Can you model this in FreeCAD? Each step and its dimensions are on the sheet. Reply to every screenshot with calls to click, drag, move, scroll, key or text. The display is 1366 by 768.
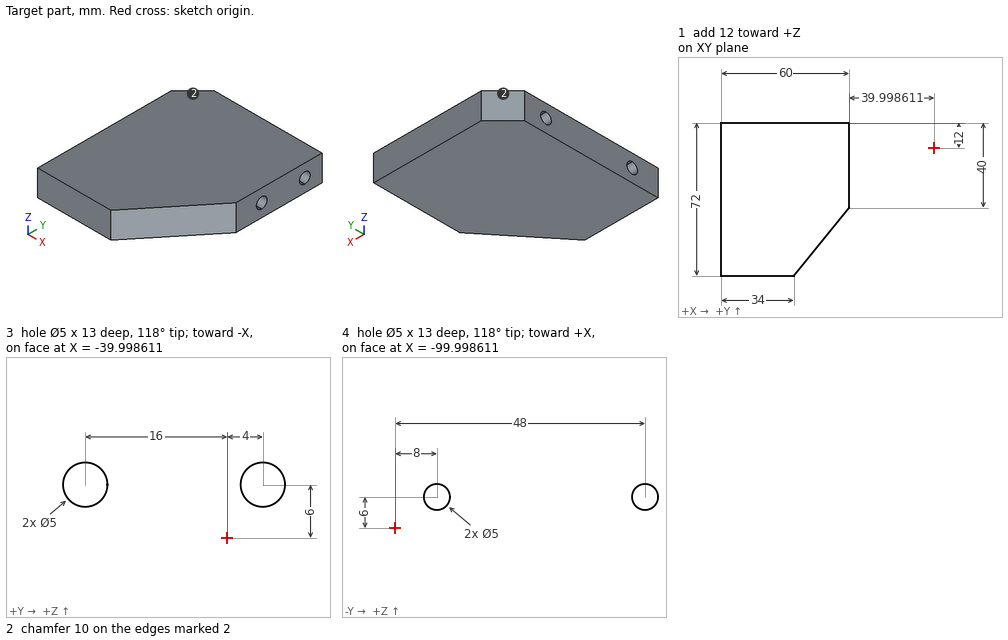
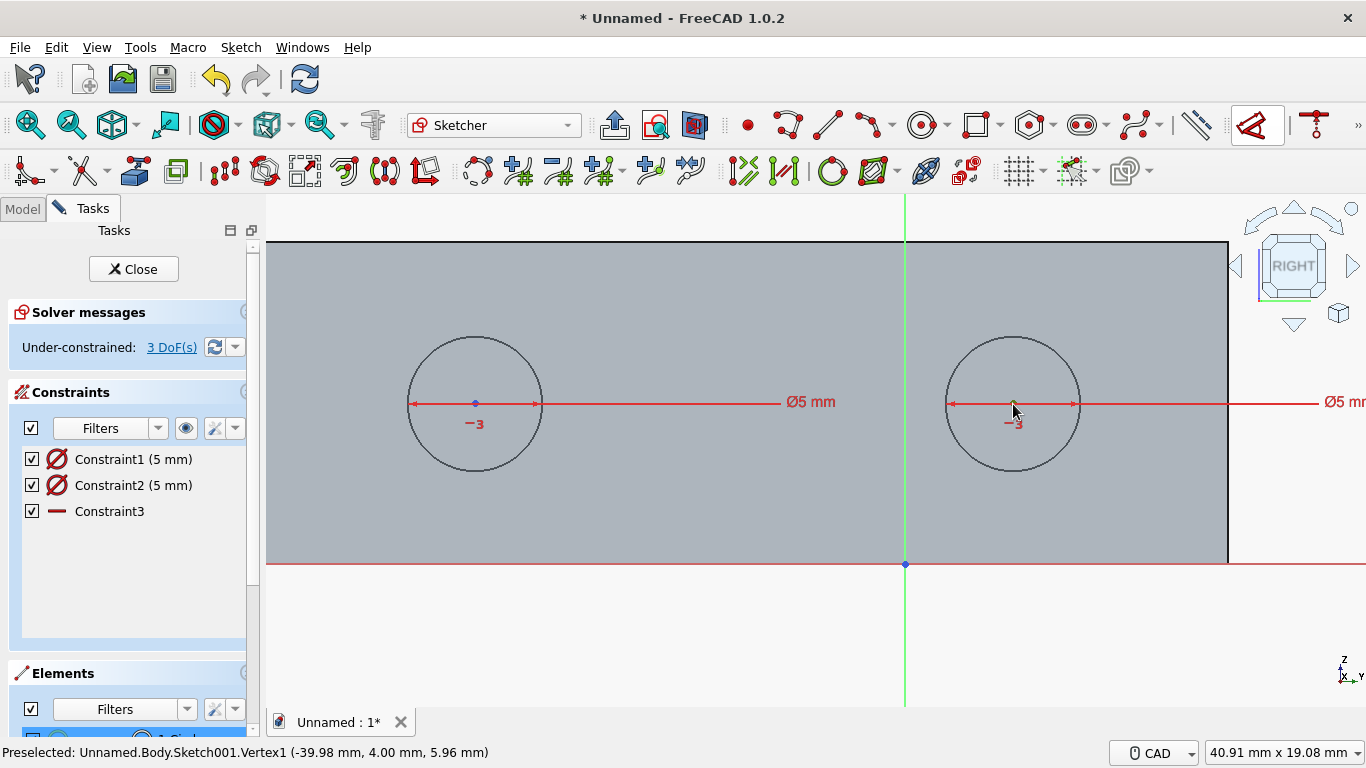
click(1278, 126)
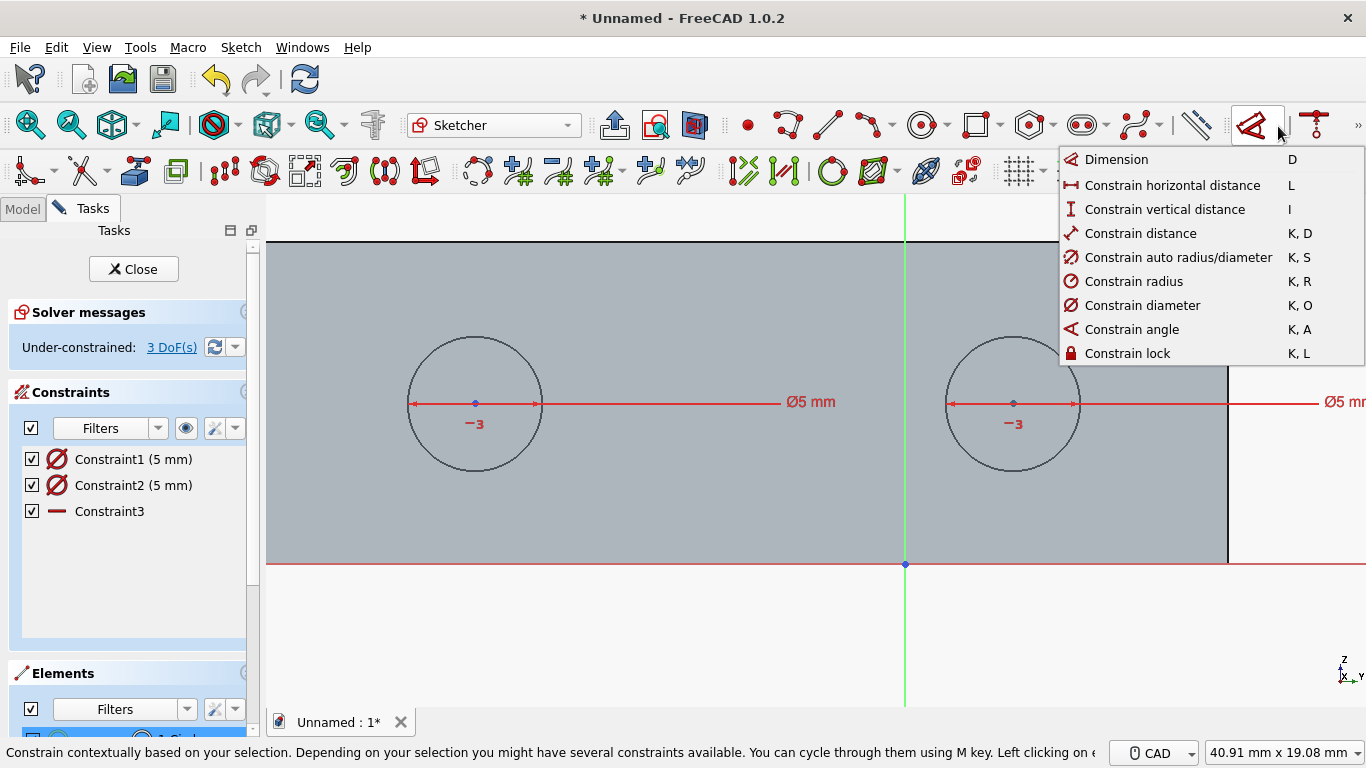
click(1212, 185)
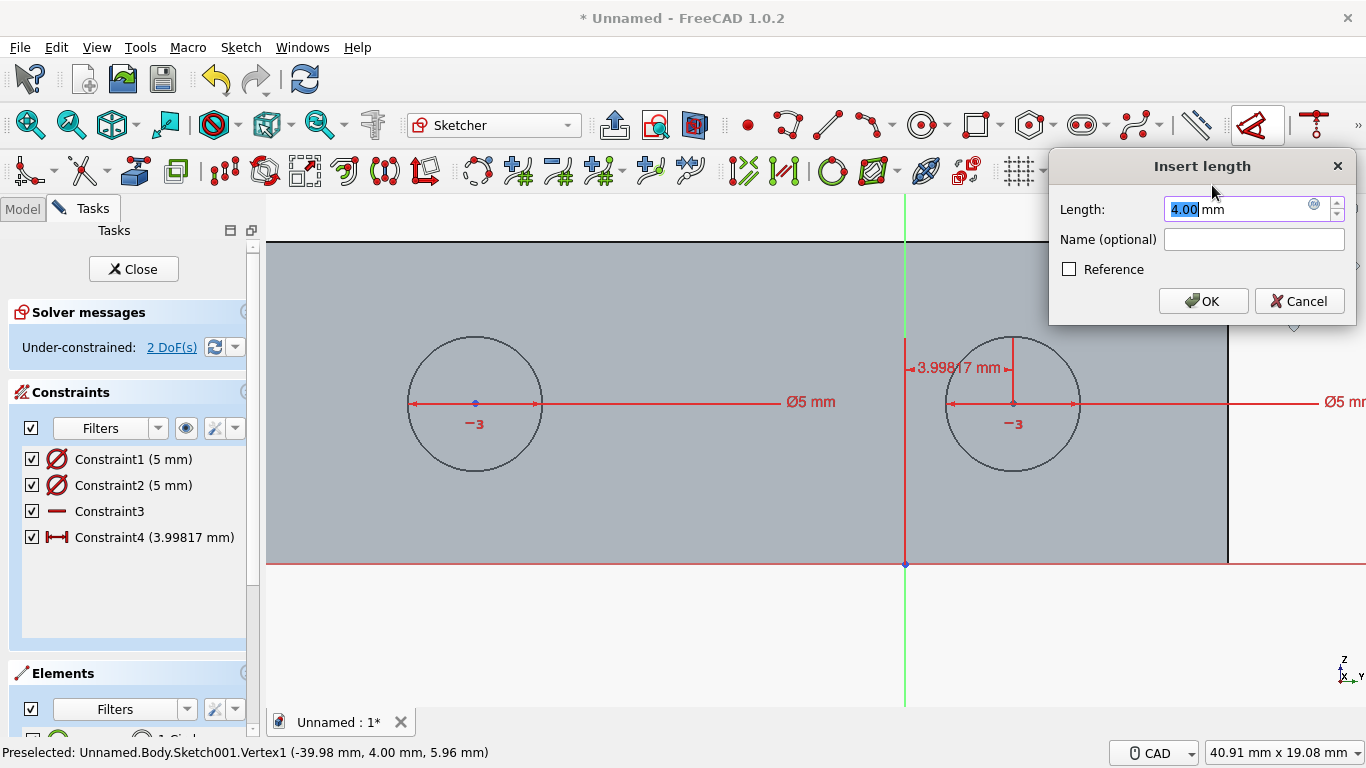
text(4)
key(Return)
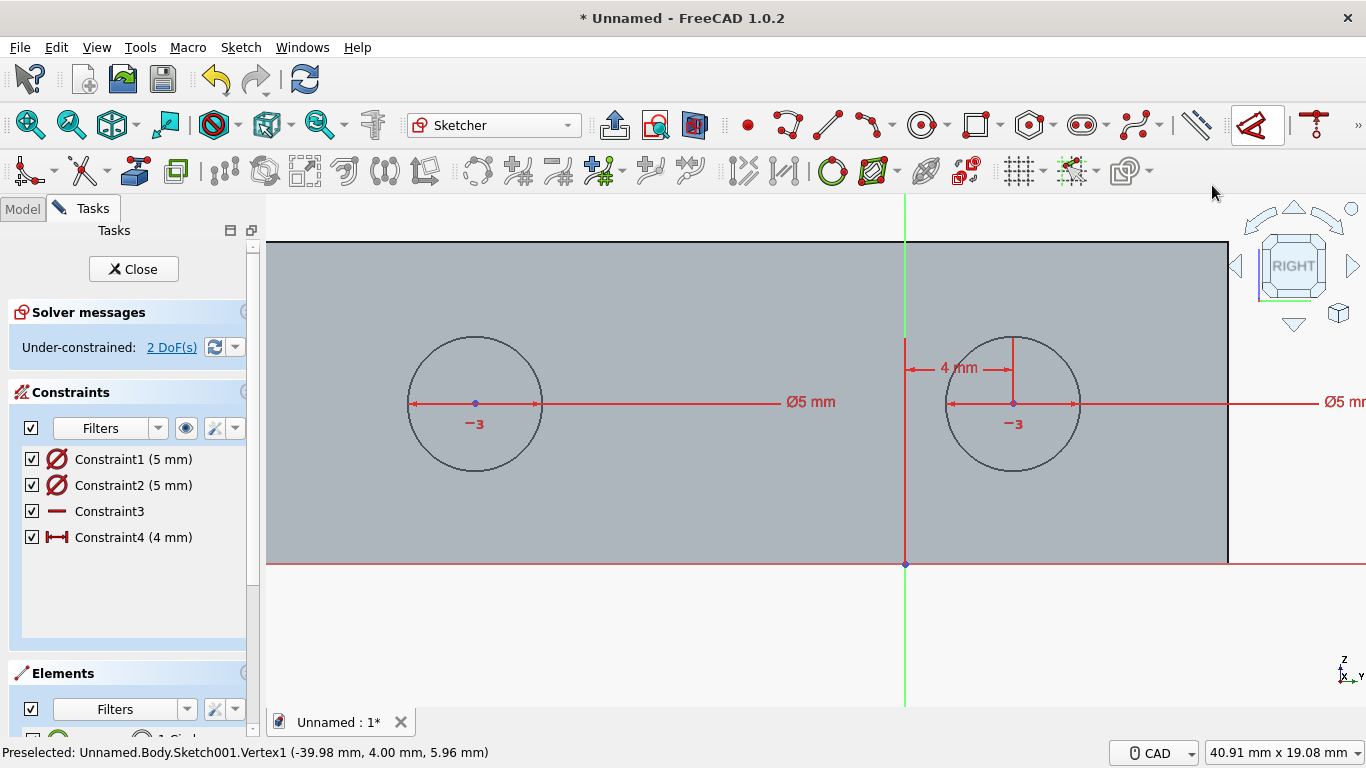
click(1013, 404)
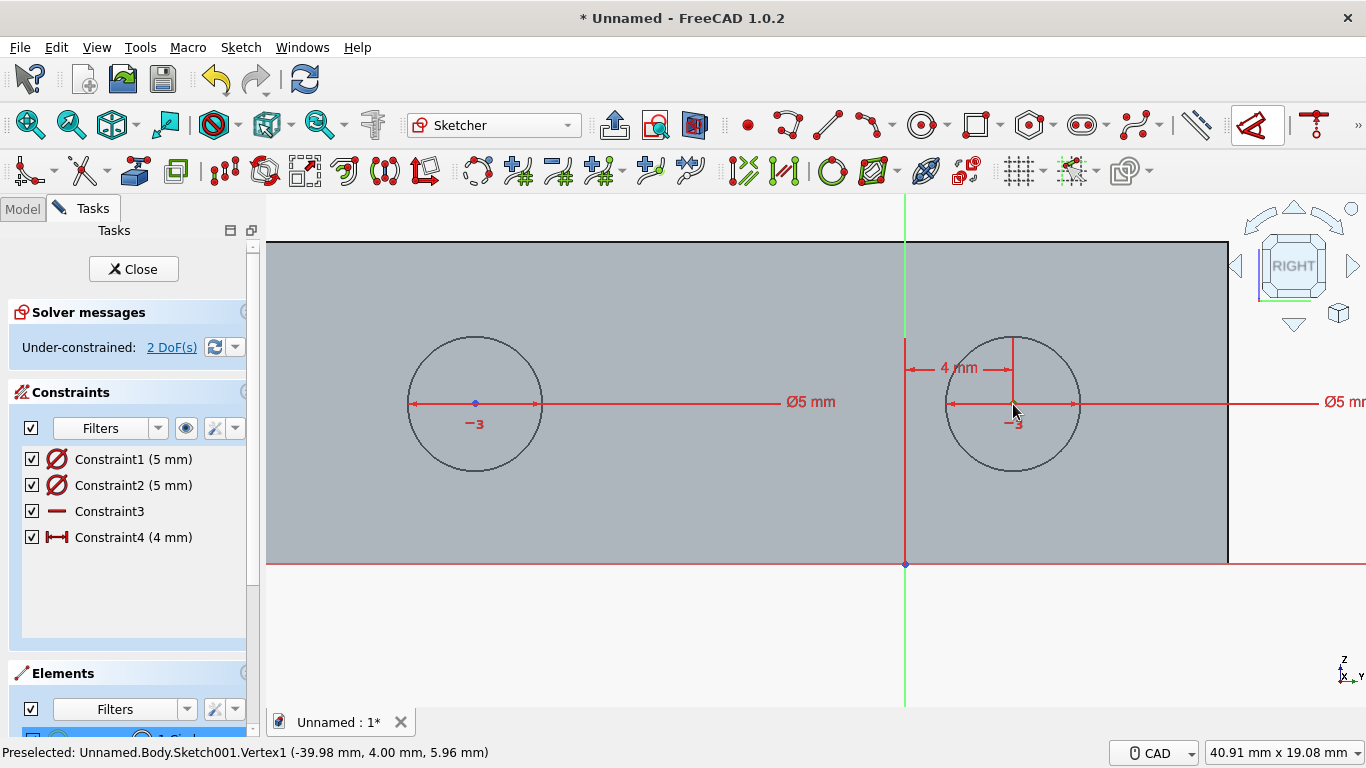
click(1278, 126)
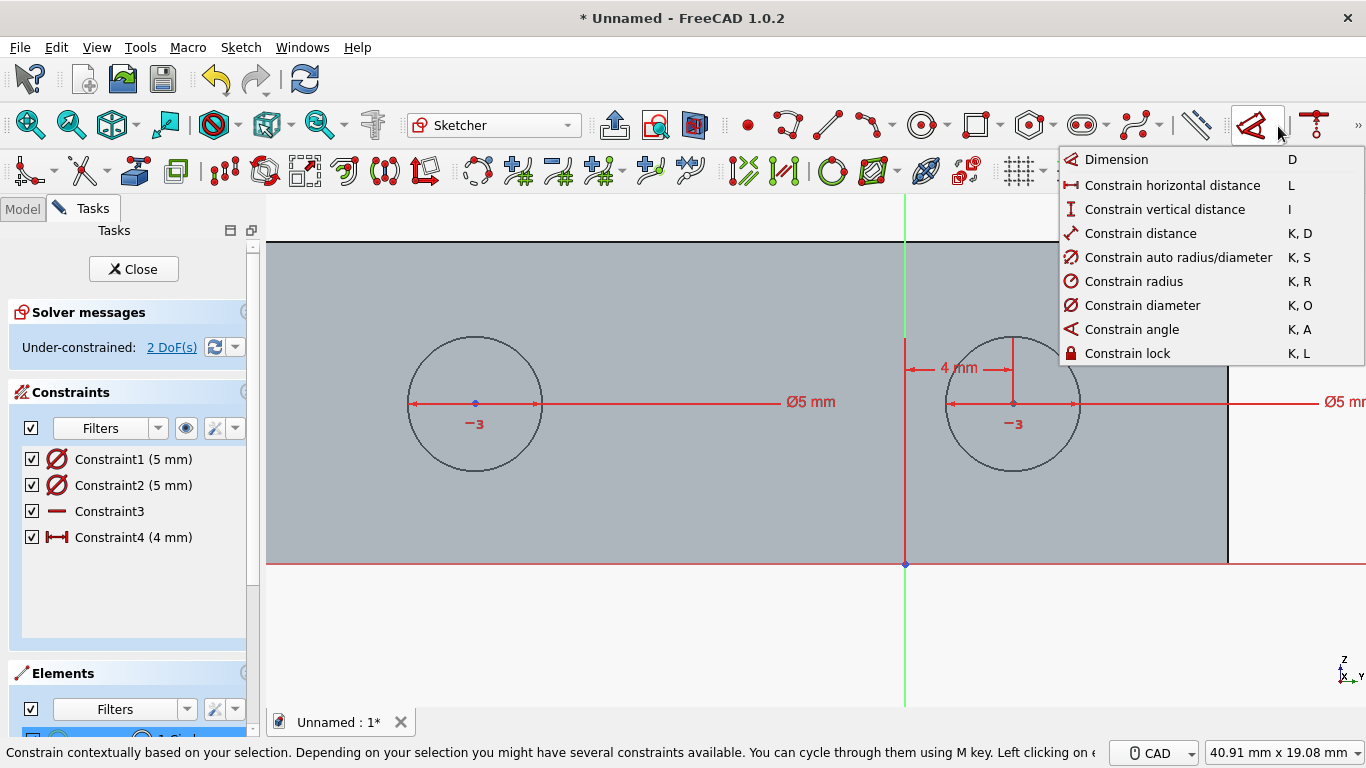
click(1212, 209)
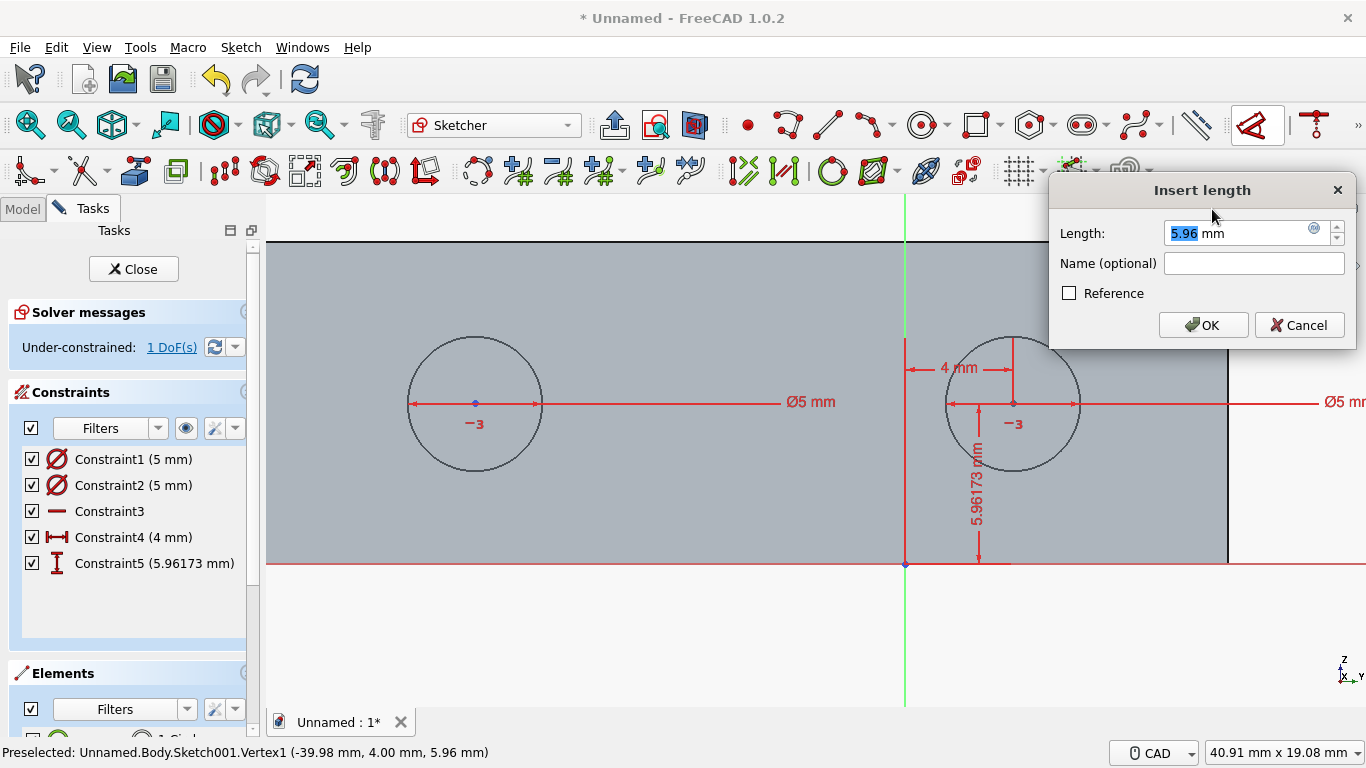
text(6)
key(Return)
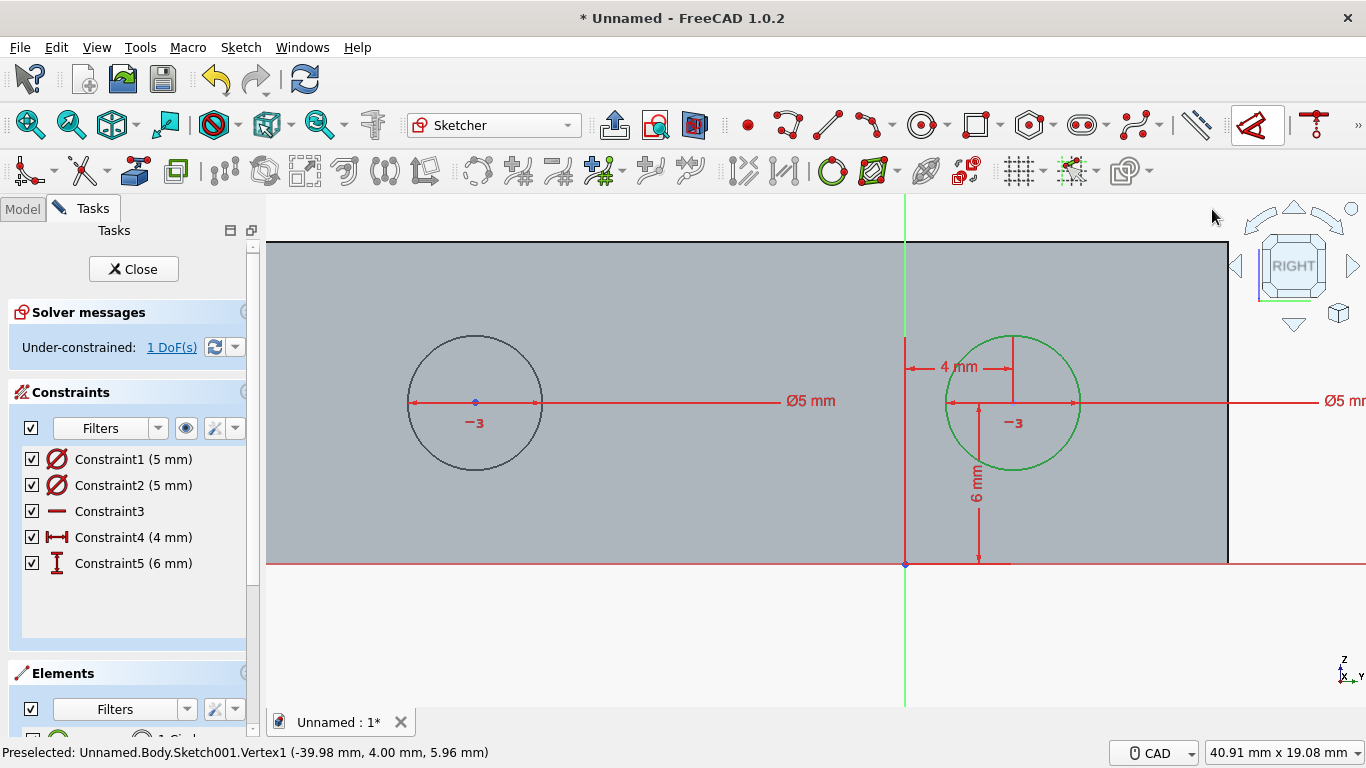
click(475, 403)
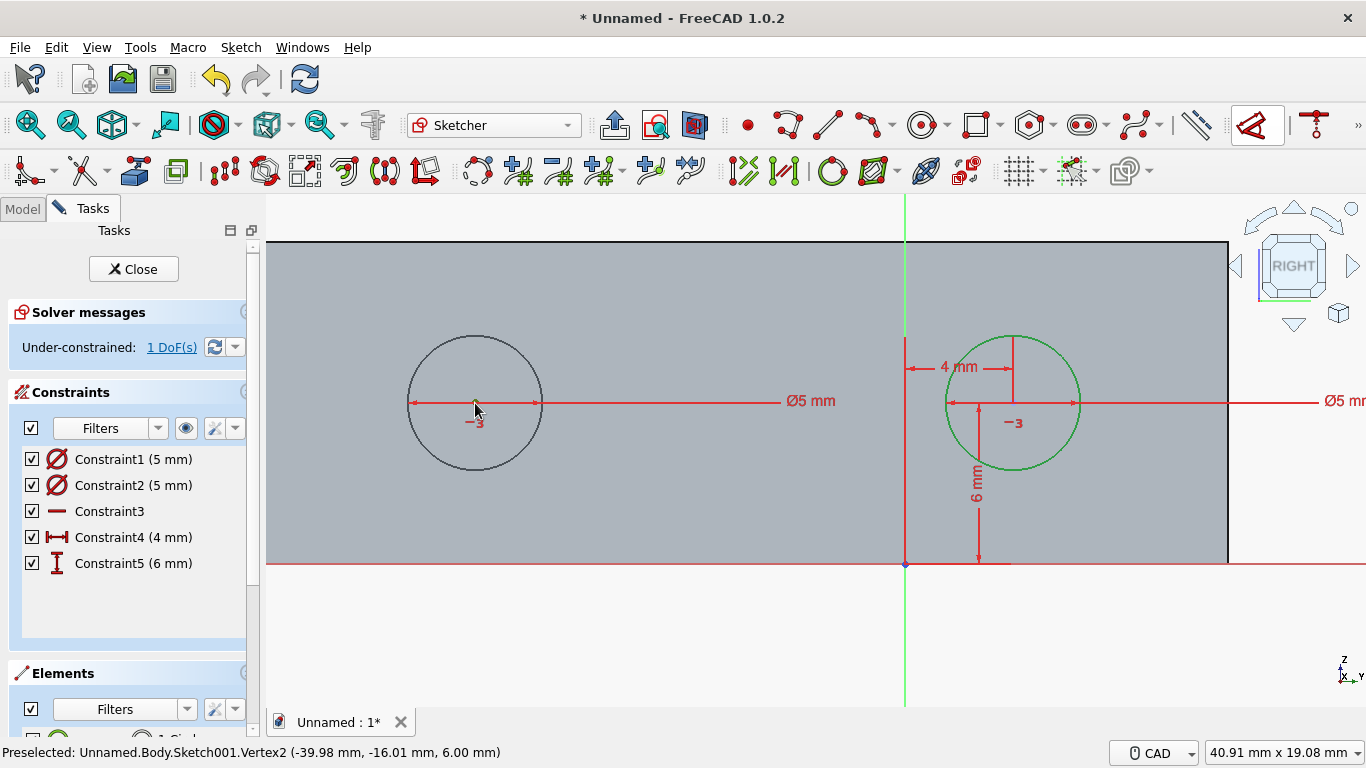
click(1278, 126)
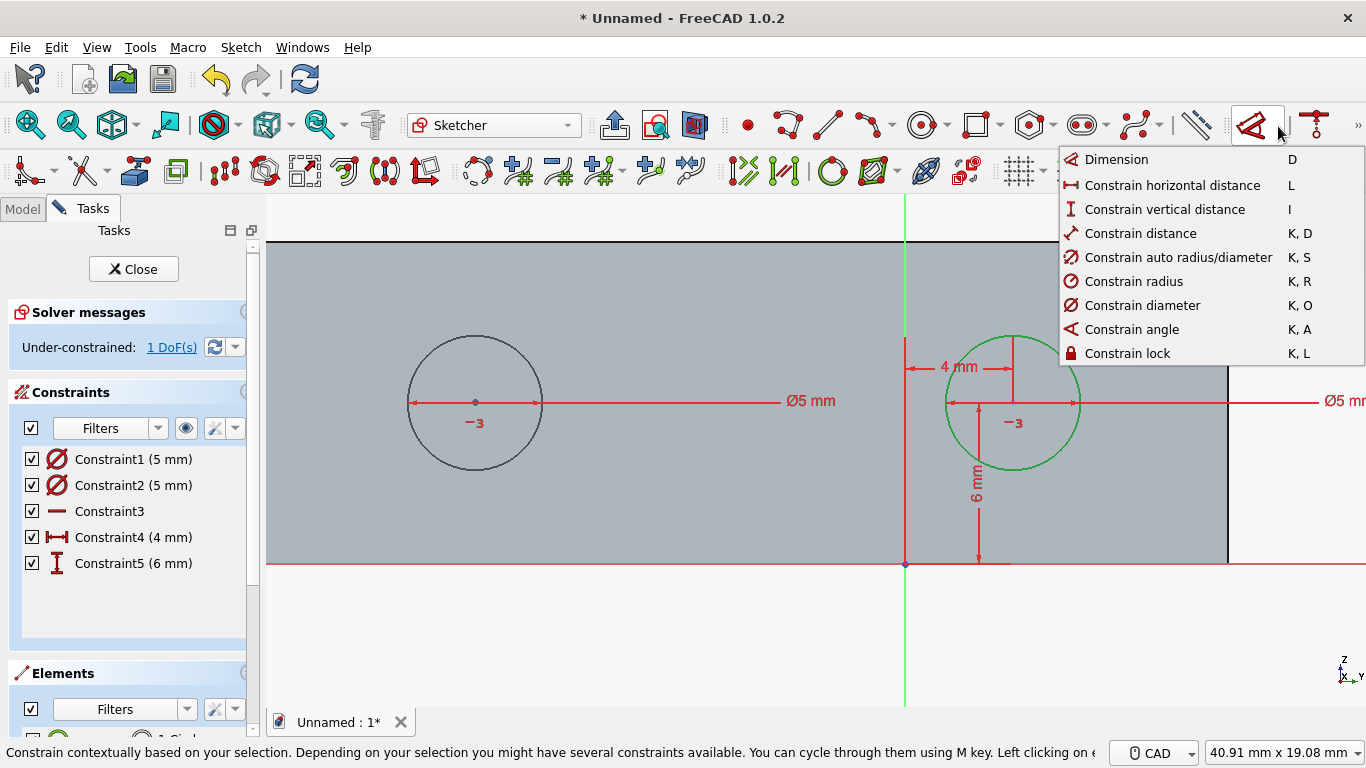
click(1212, 185)